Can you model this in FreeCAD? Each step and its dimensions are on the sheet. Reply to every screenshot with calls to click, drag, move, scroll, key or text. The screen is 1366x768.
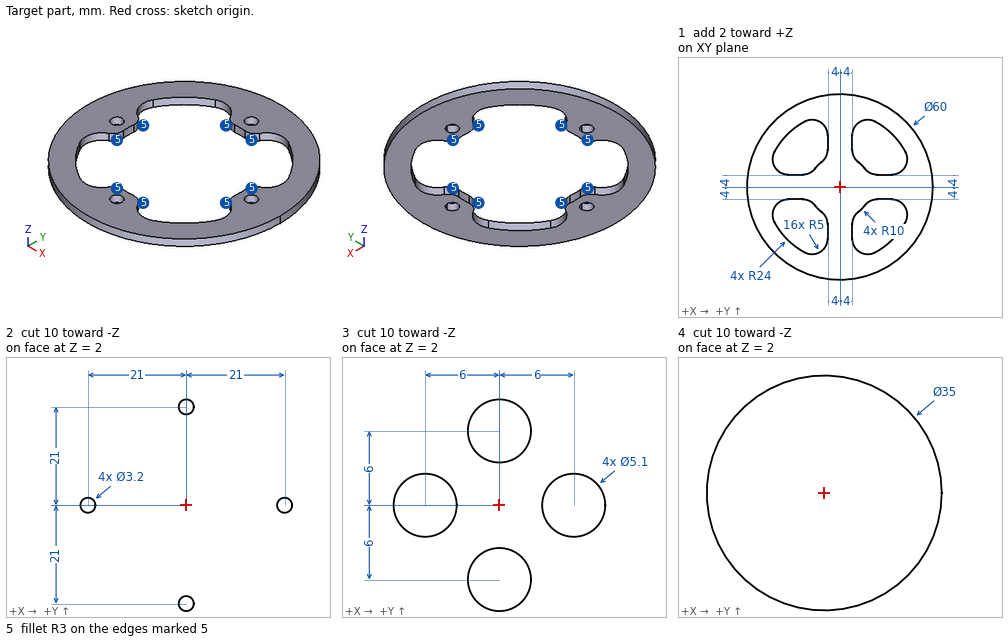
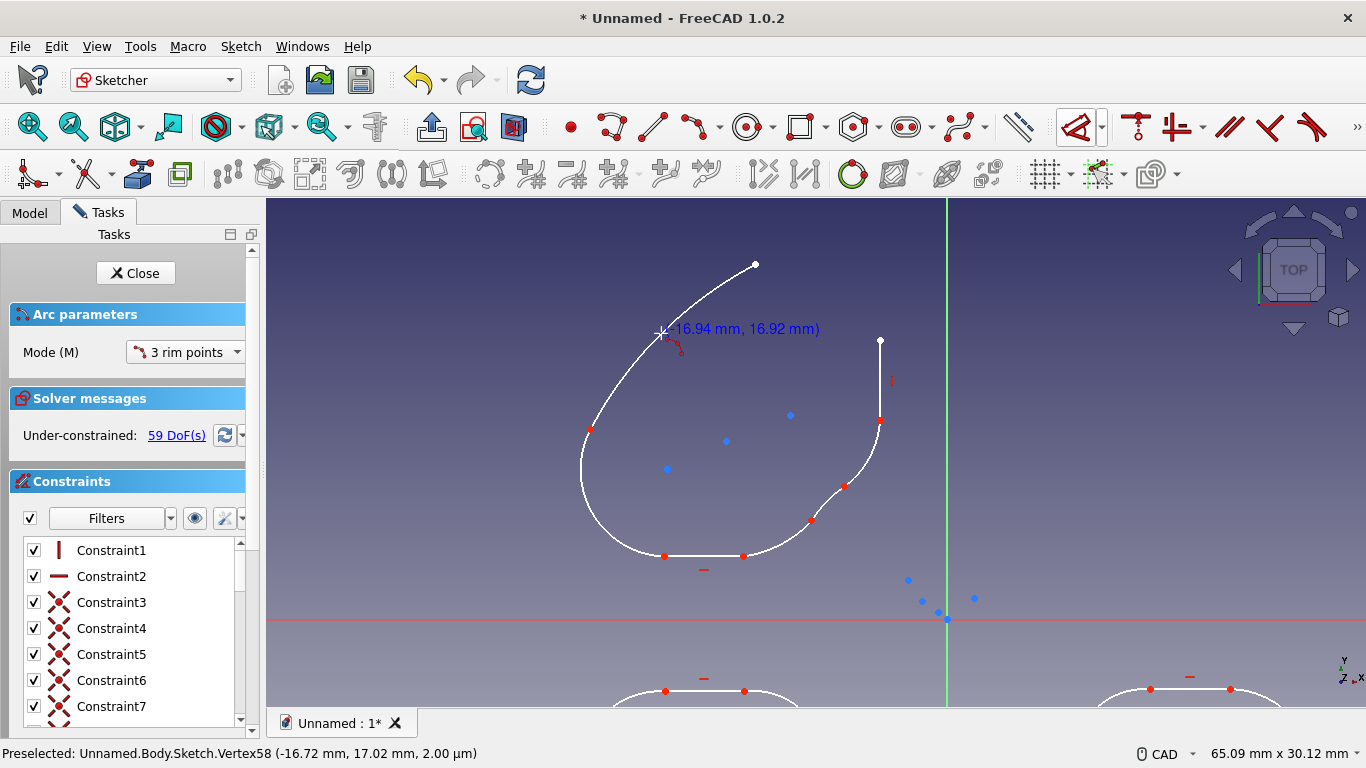
click(755, 265)
click(880, 341)
click(839, 265)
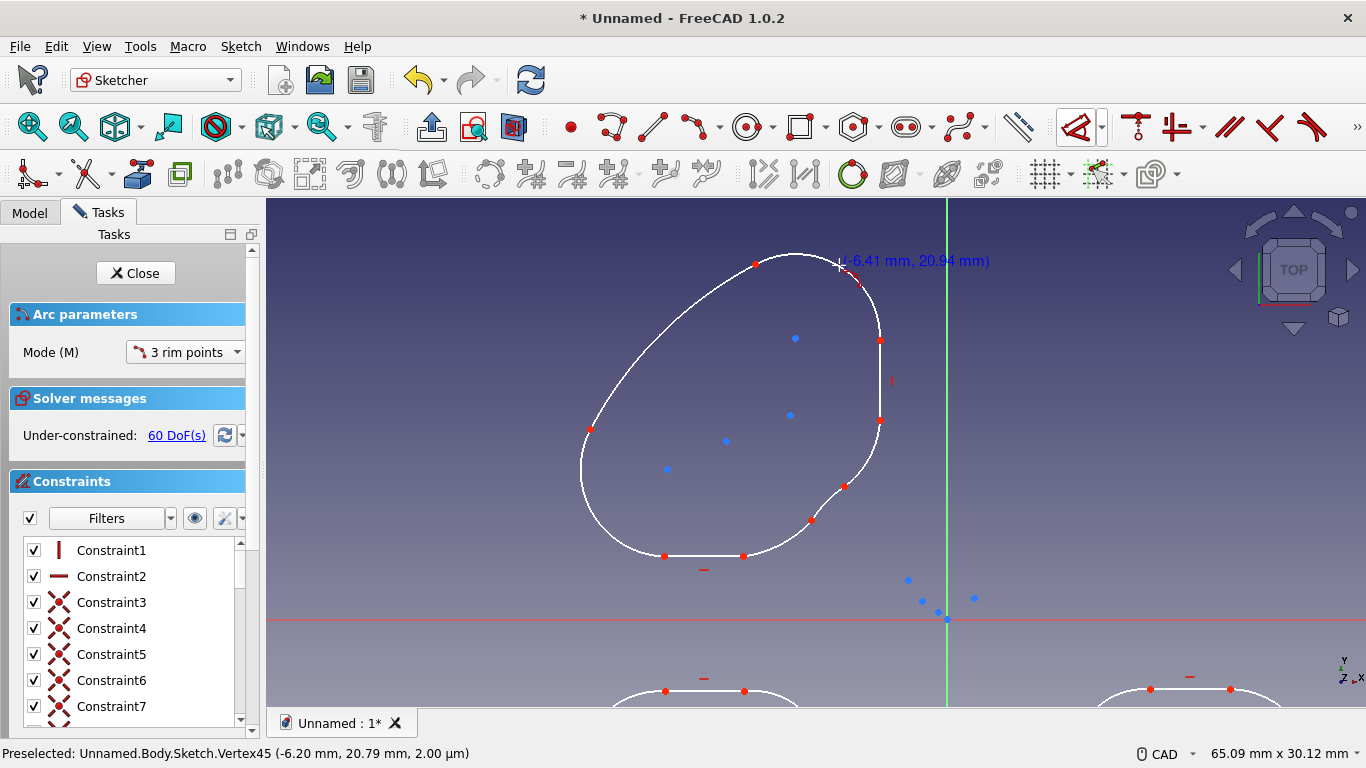
key(g)
key(l)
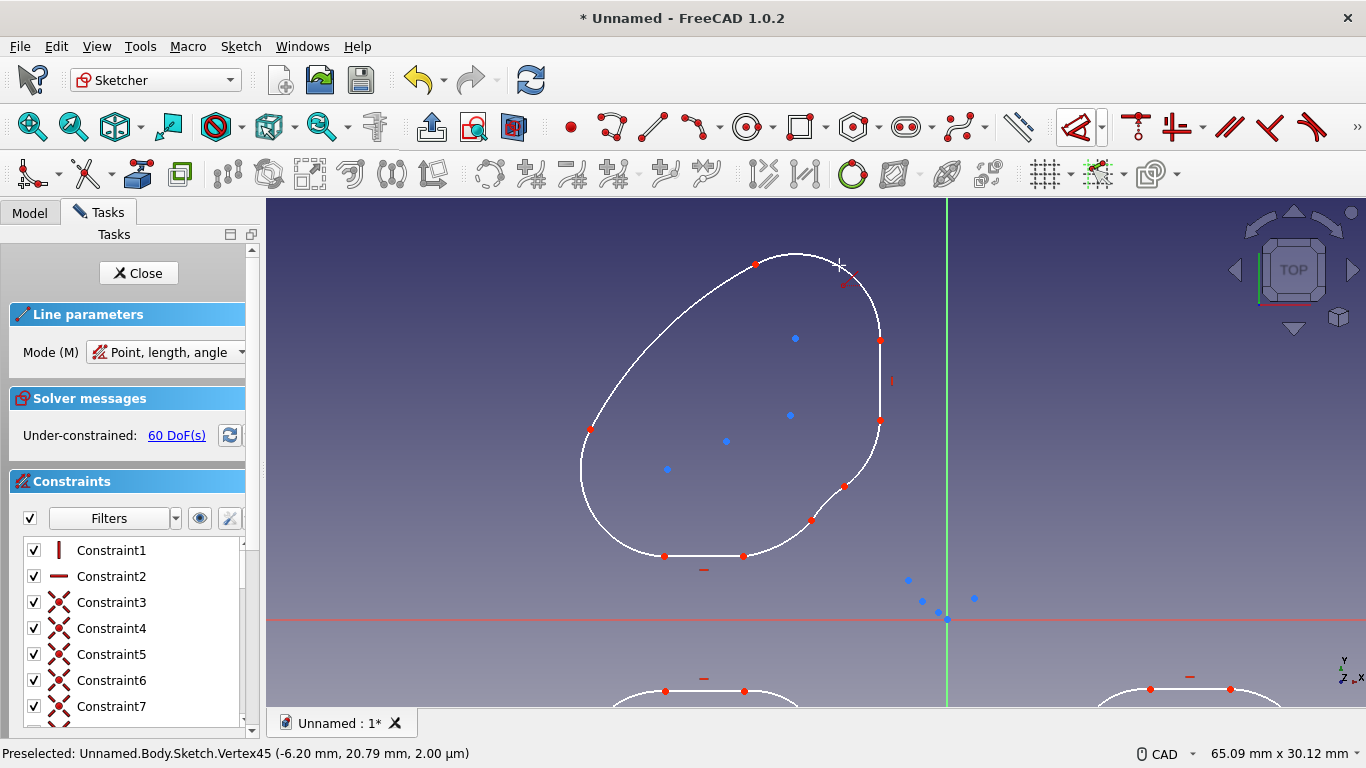
click(1015, 417)
click(1015, 337)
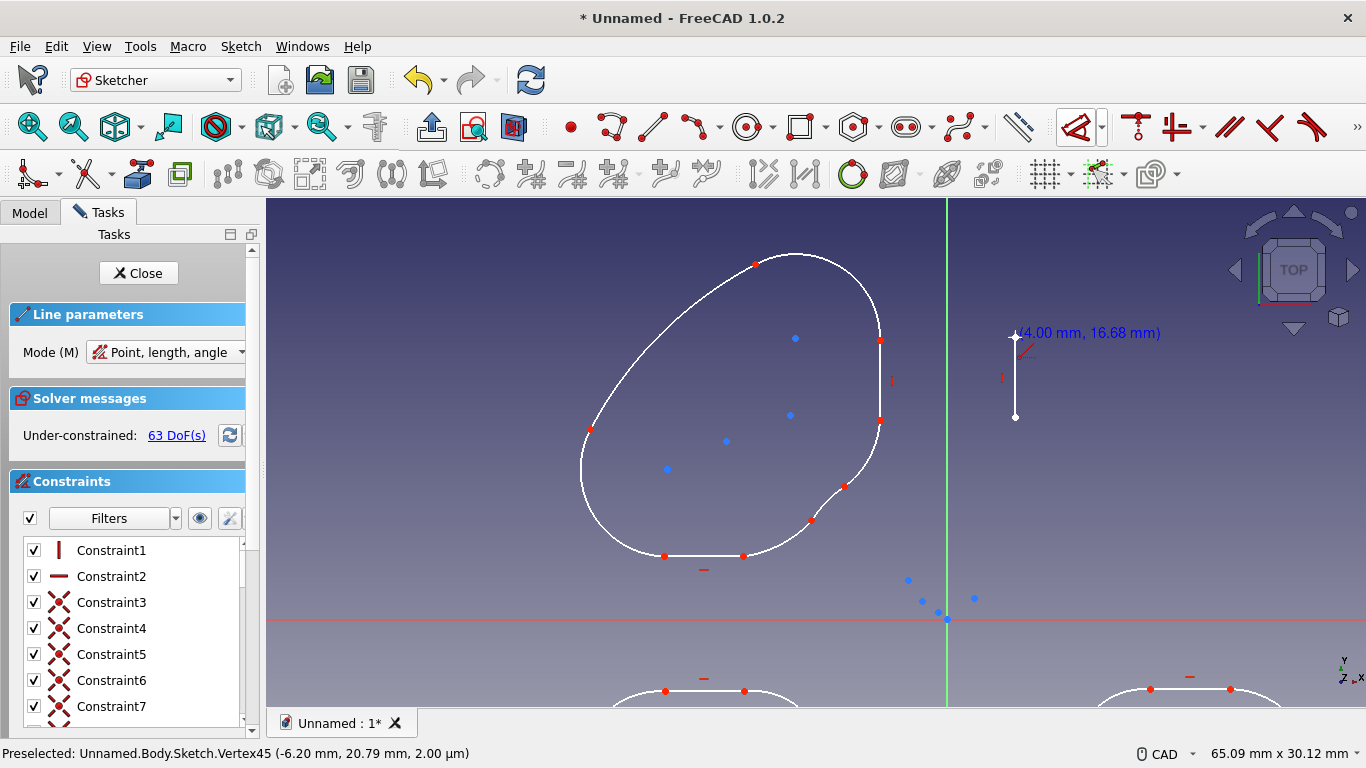
scroll(661, 380, down, 6)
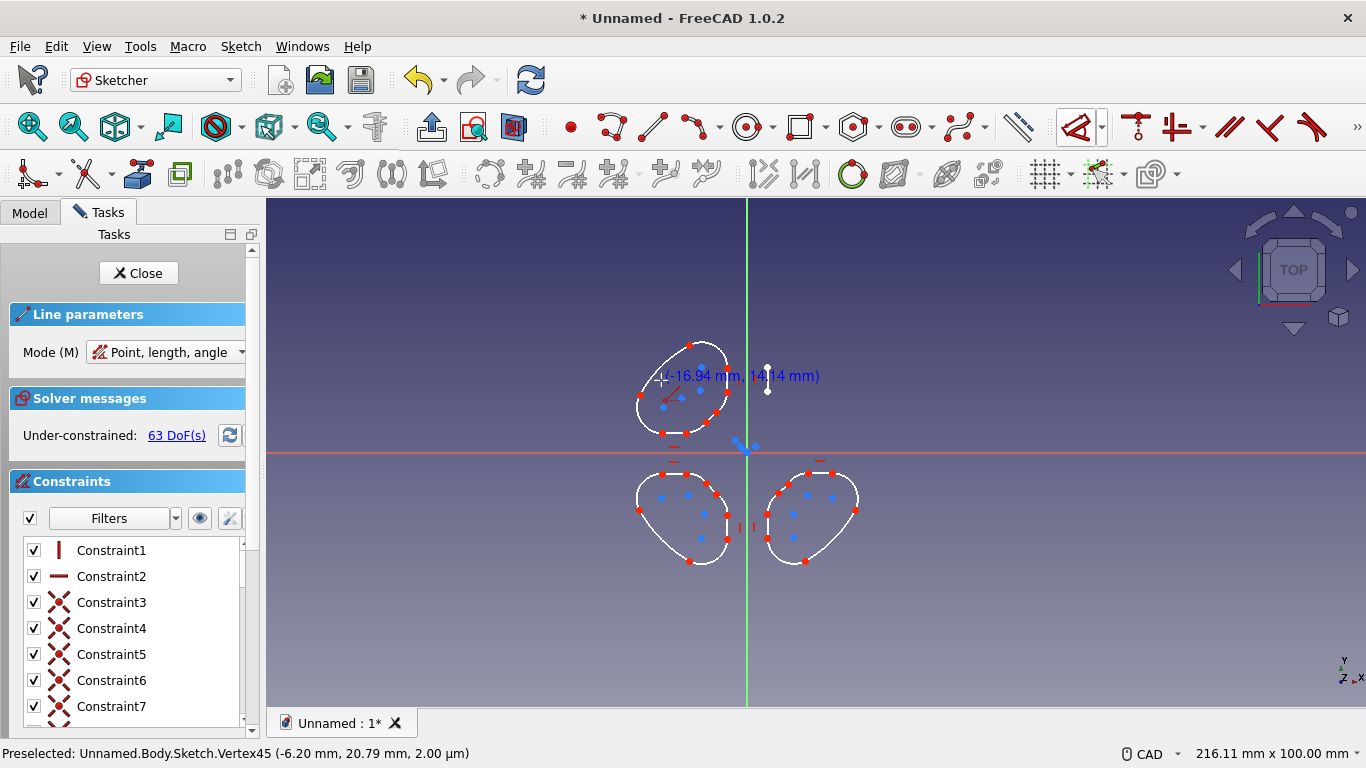
click(833, 432)
click(809, 432)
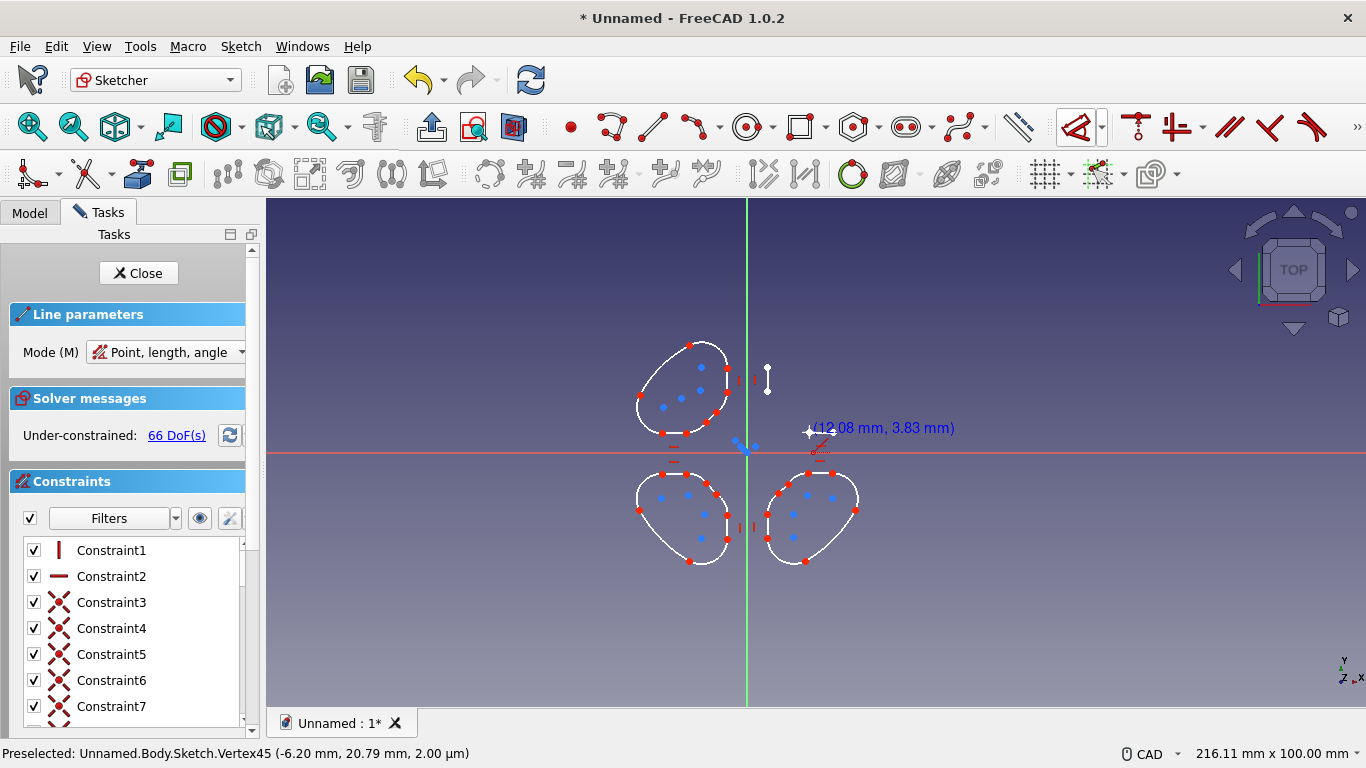
key(g)
key(3)
key(a)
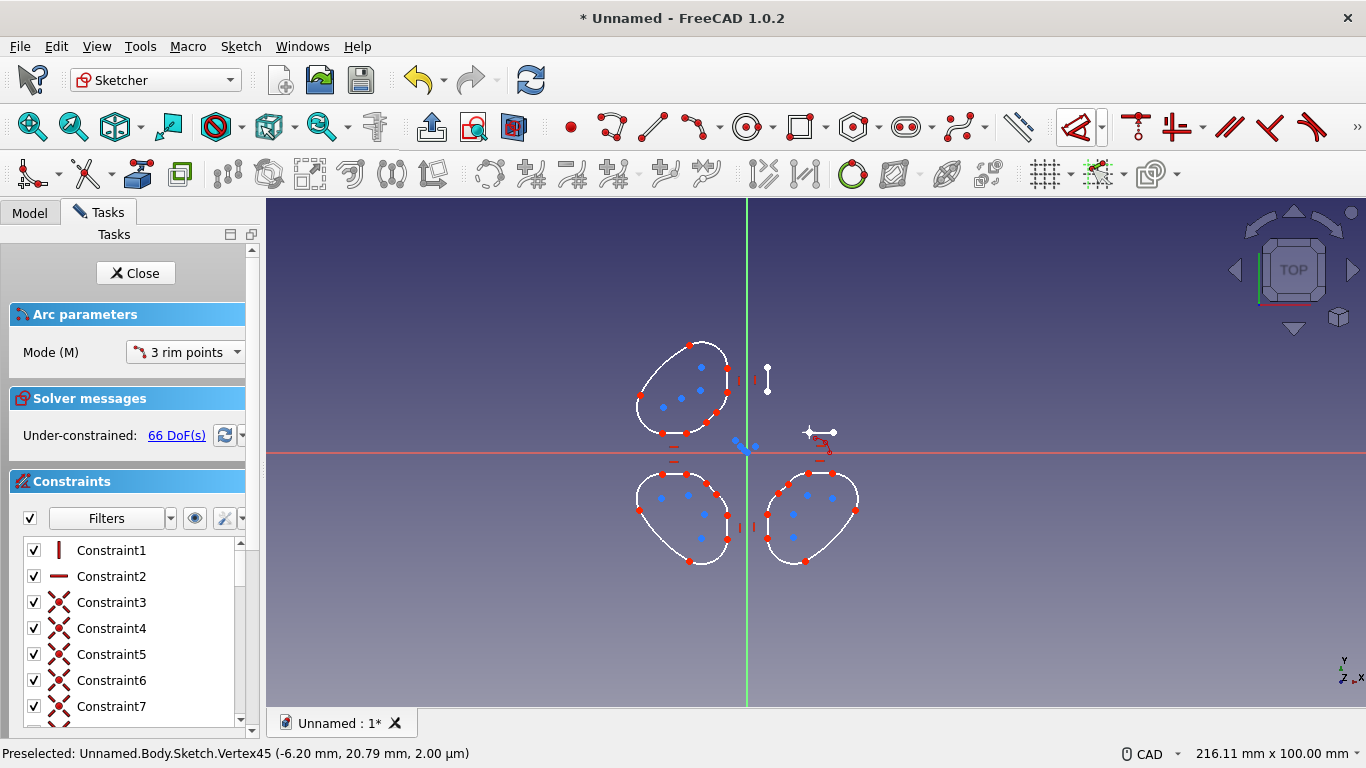
scroll(768, 367, up, 2)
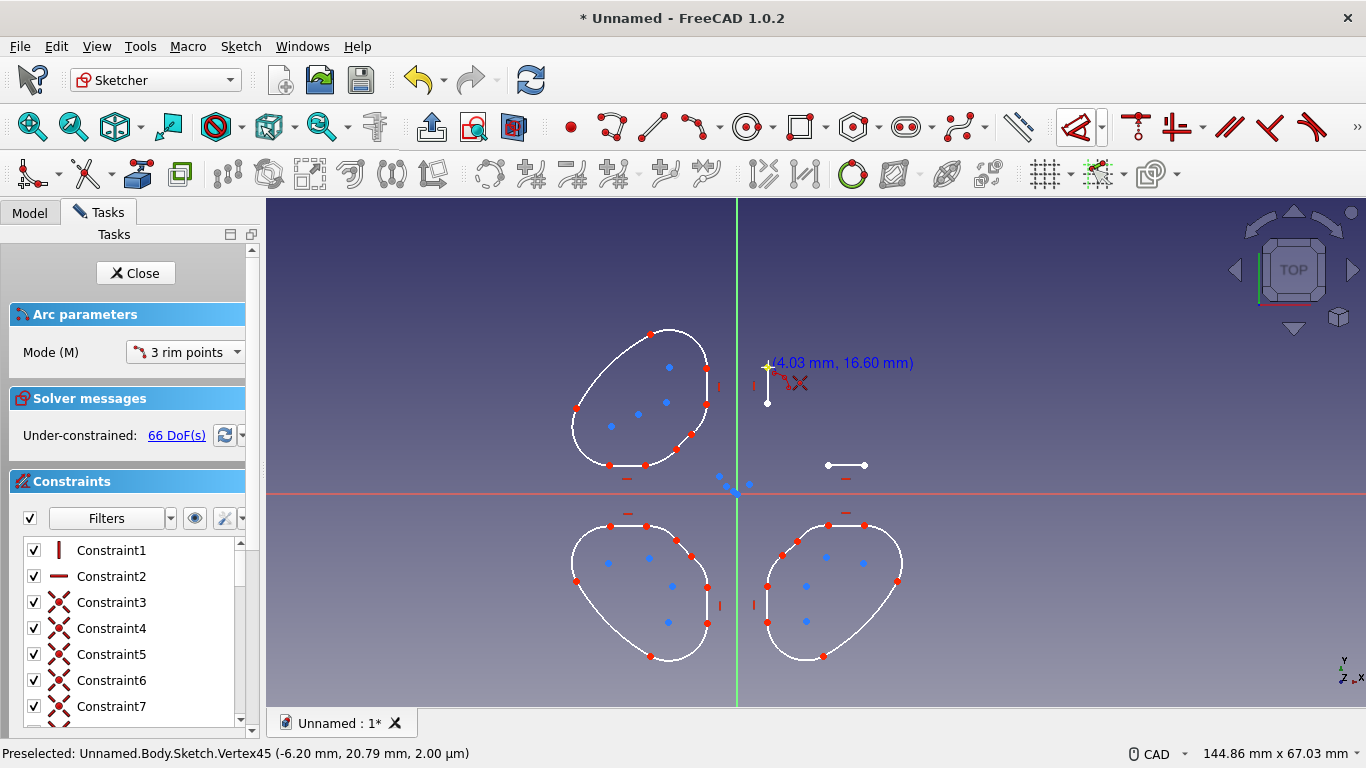
click(768, 368)
click(824, 334)
click(786, 335)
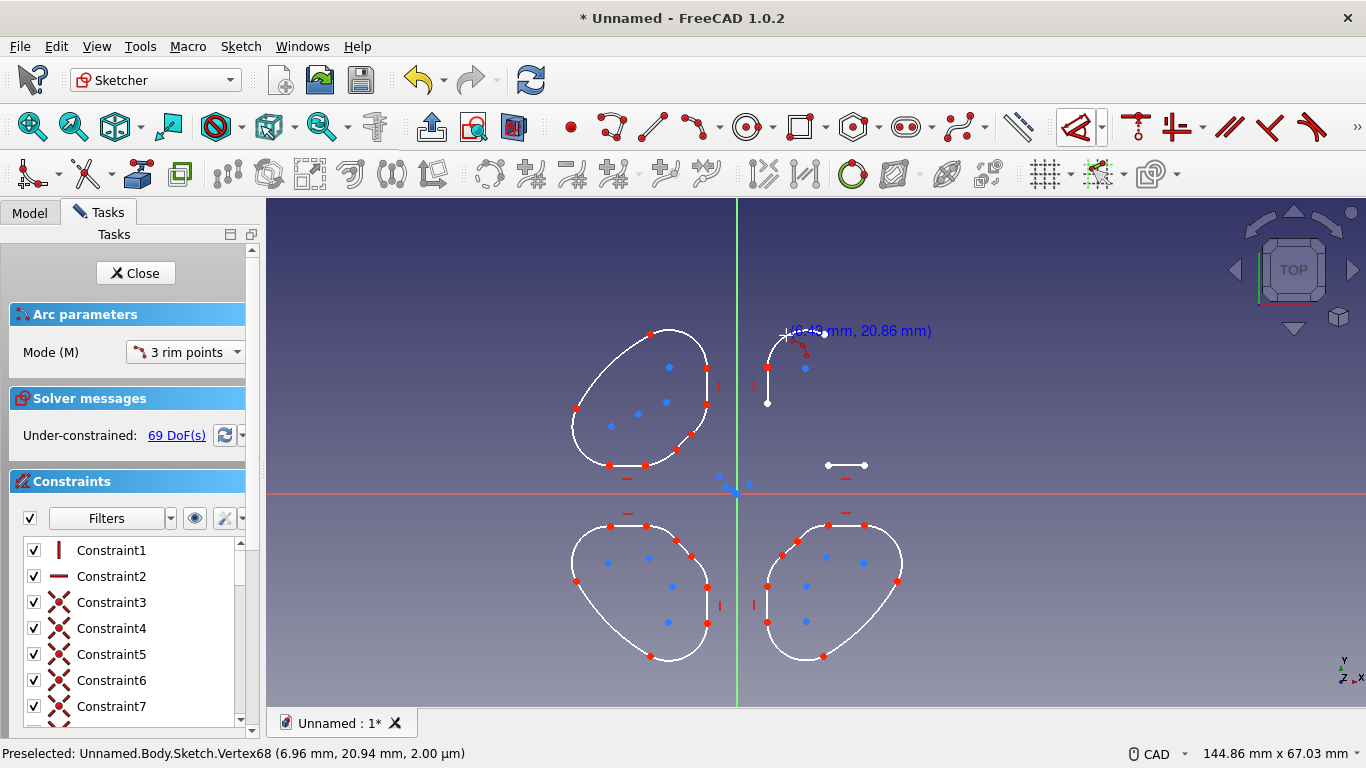
click(824, 335)
click(898, 408)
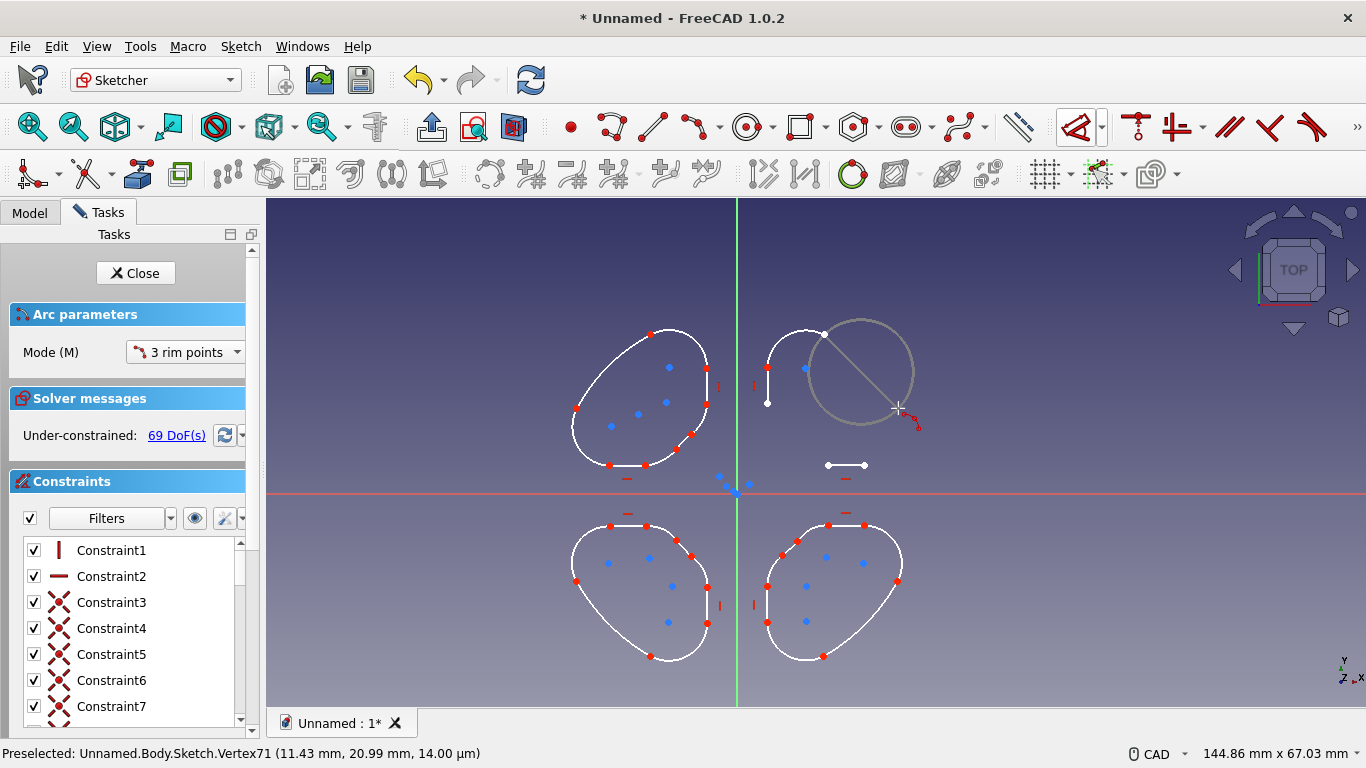
scroll(866, 366, up, 4)